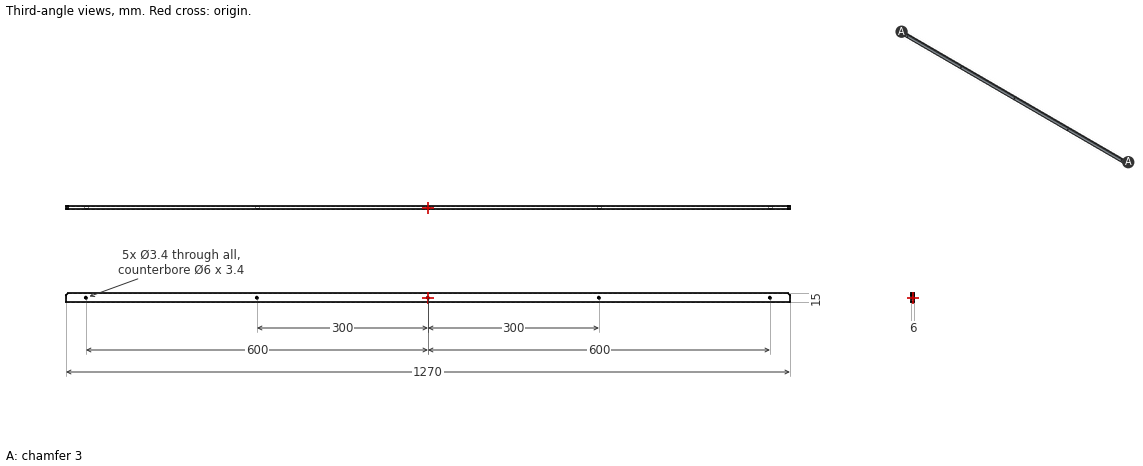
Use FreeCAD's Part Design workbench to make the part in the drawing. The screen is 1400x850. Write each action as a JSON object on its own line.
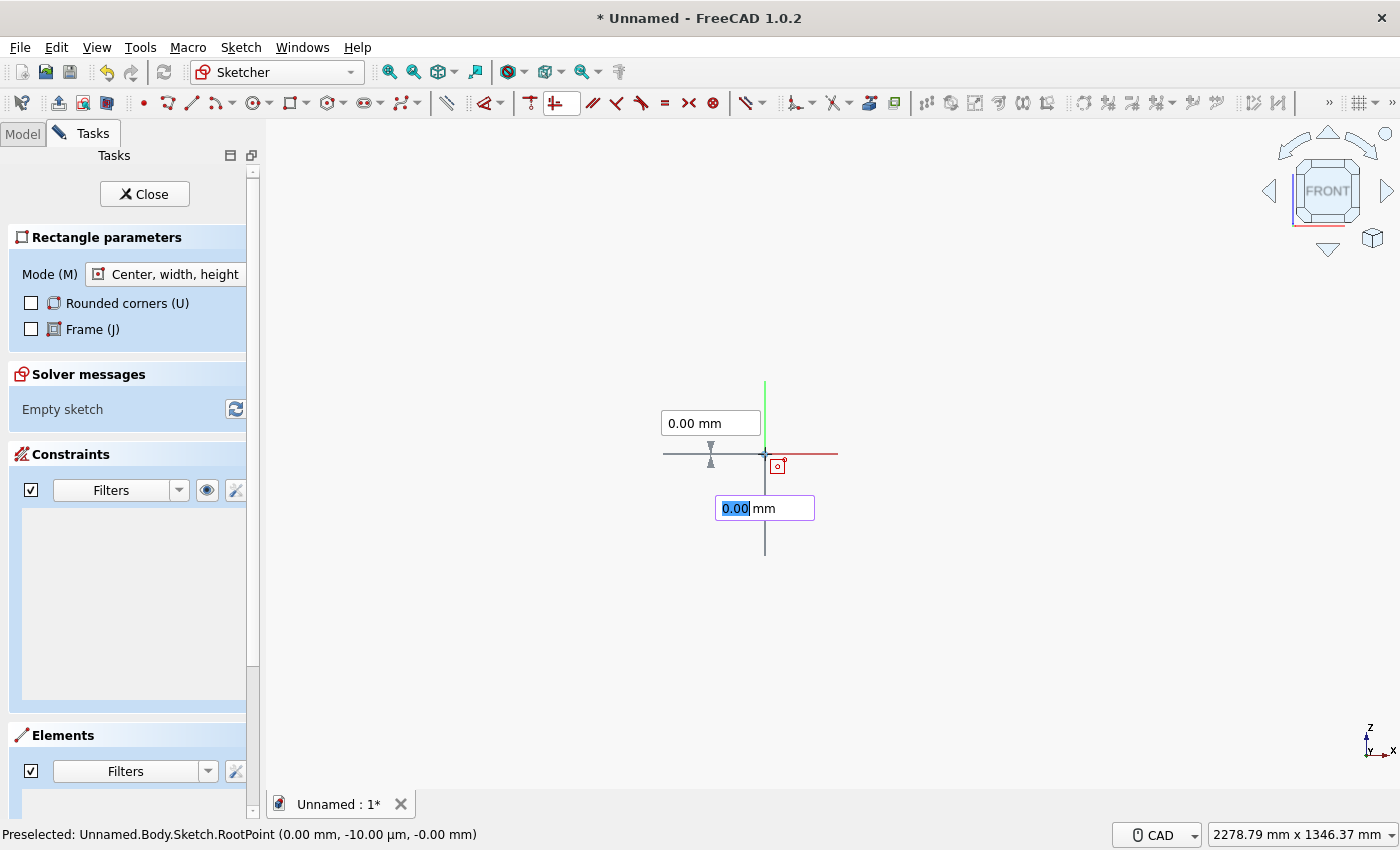
{"action": "scroll", "coordinate": [1081, 451], "scroll_direction": "up", "scroll_amount": 8}
{"action": "mouse_move", "coordinate": [1078, 448]}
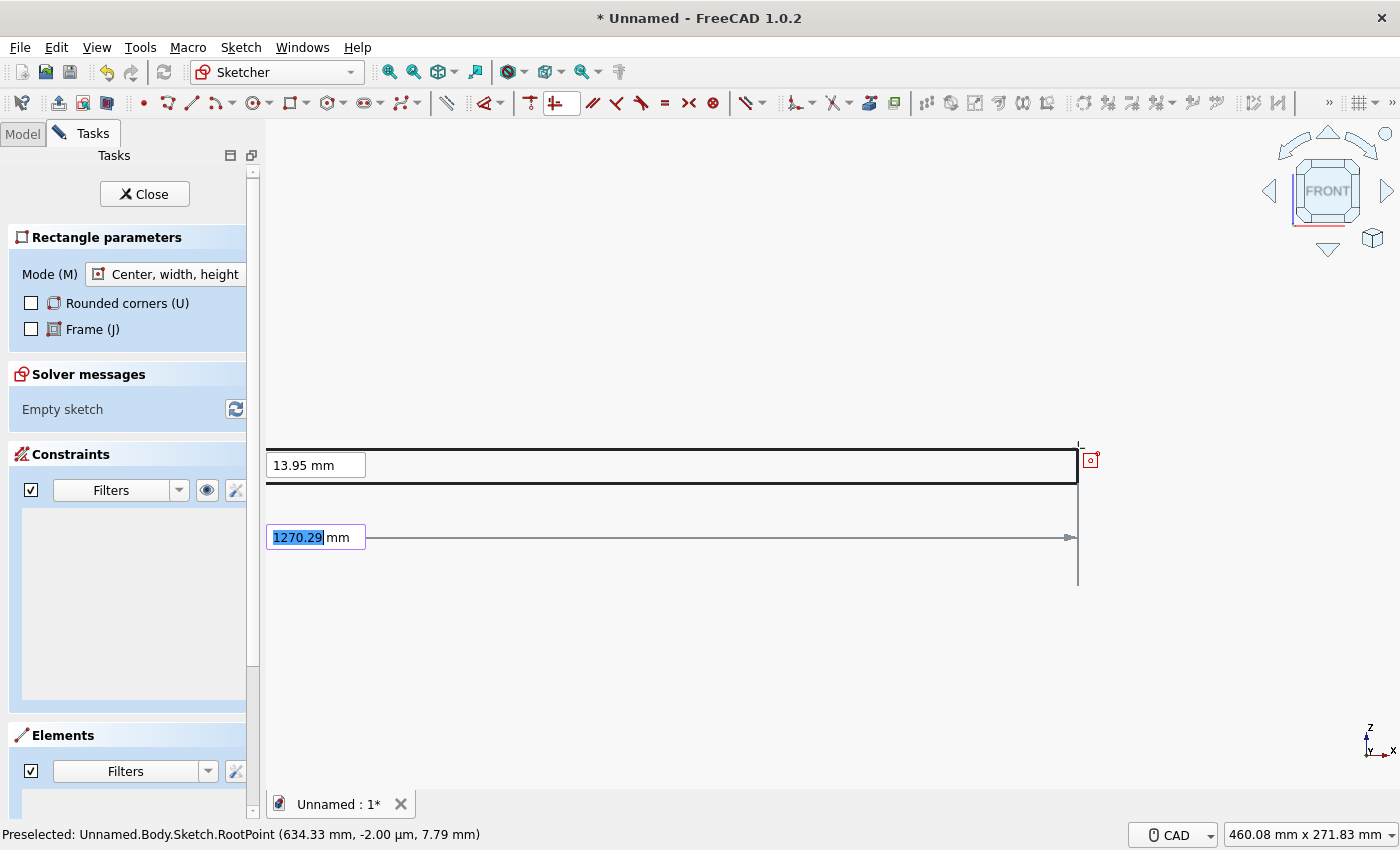
{"action": "type", "text": "1270"}
{"action": "key", "text": "Tab"}
{"action": "type", "text": "15"}
{"action": "key", "text": "Return"}
{"action": "key", "text": "Escape"}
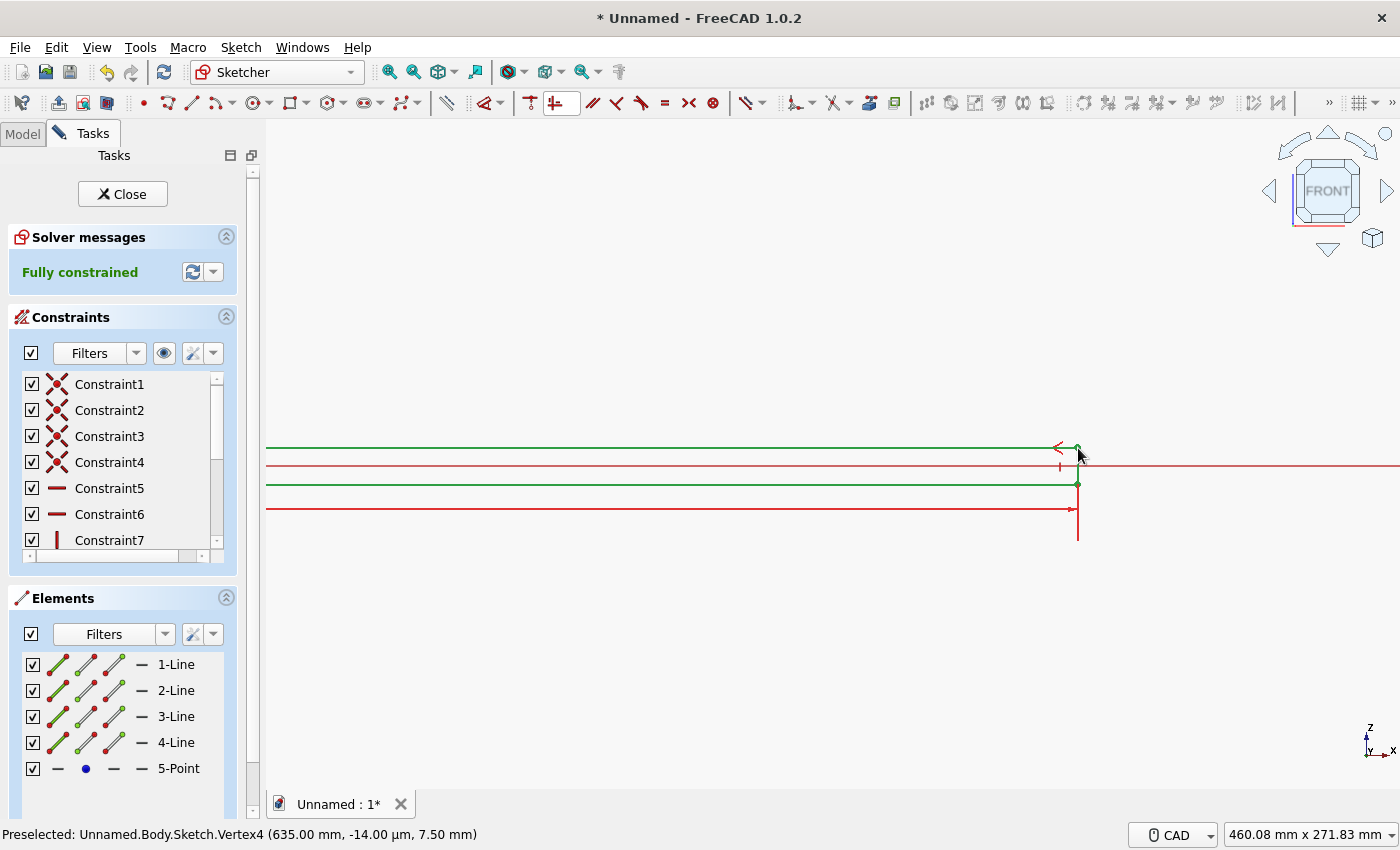
{"action": "left_click", "coordinate": [123, 194]}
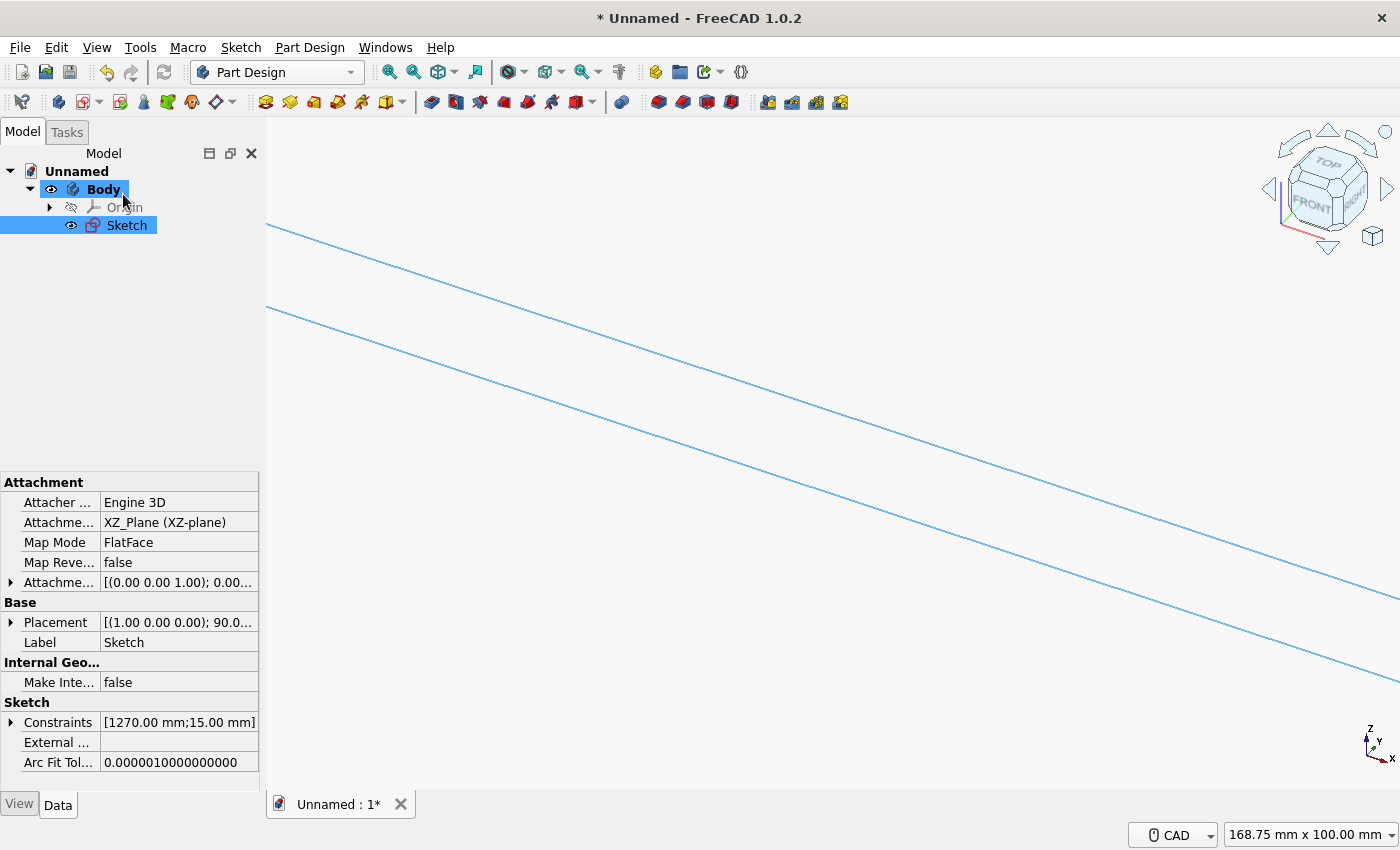
{"action": "left_click", "coordinate": [266, 102]}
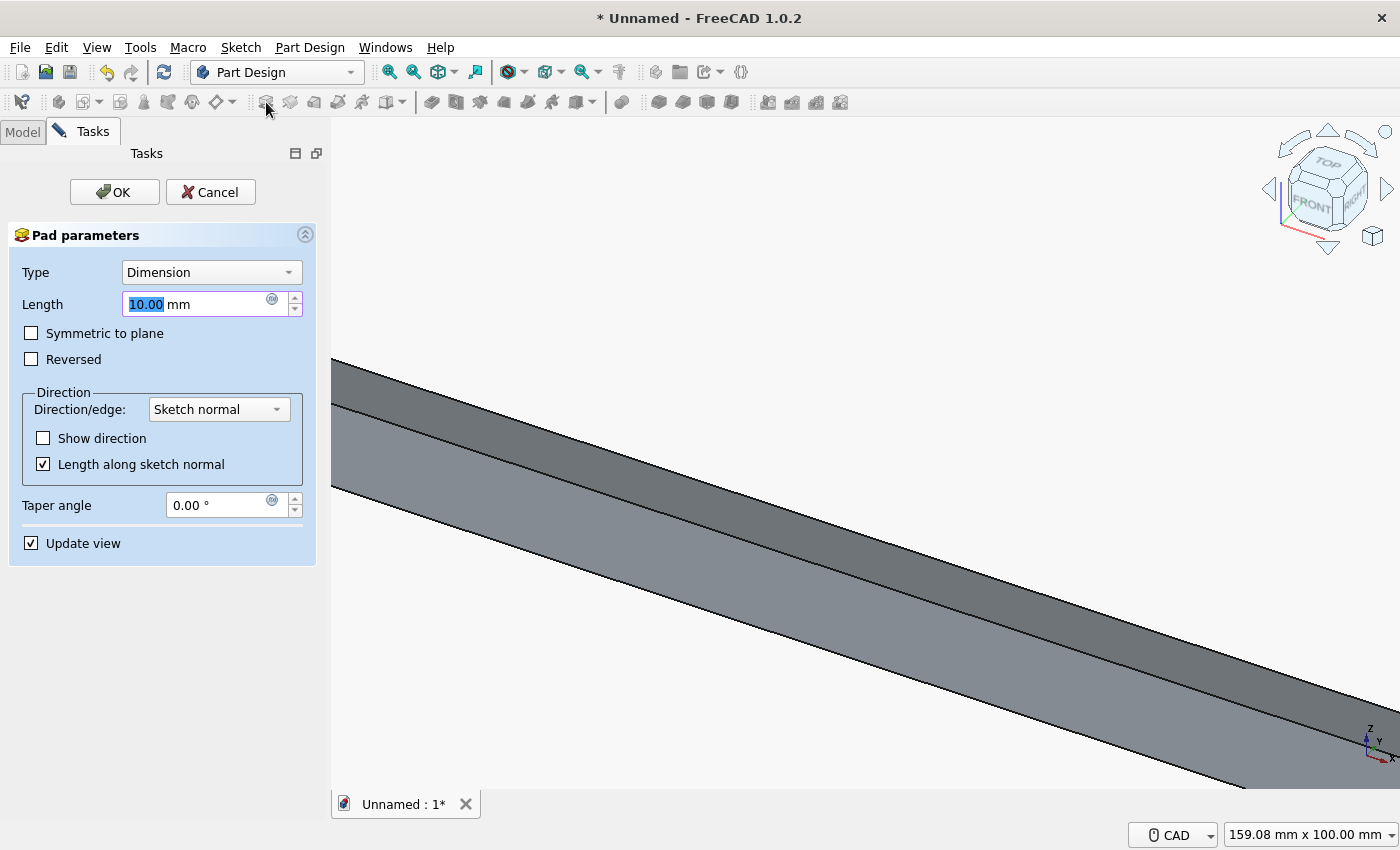
{"action": "type", "text": "6"}
{"action": "key", "text": "Tab"}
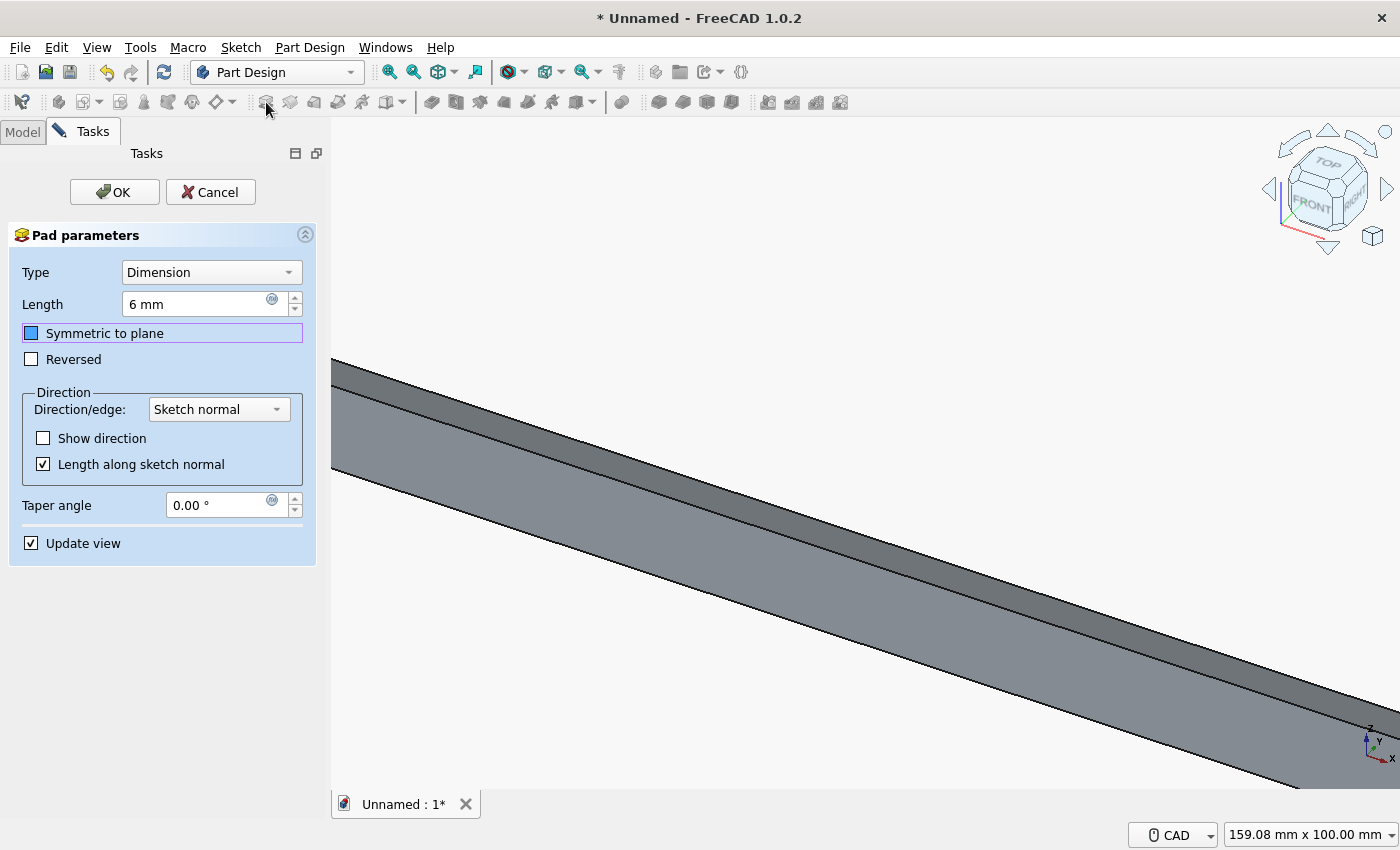
{"action": "left_click", "coordinate": [30, 333]}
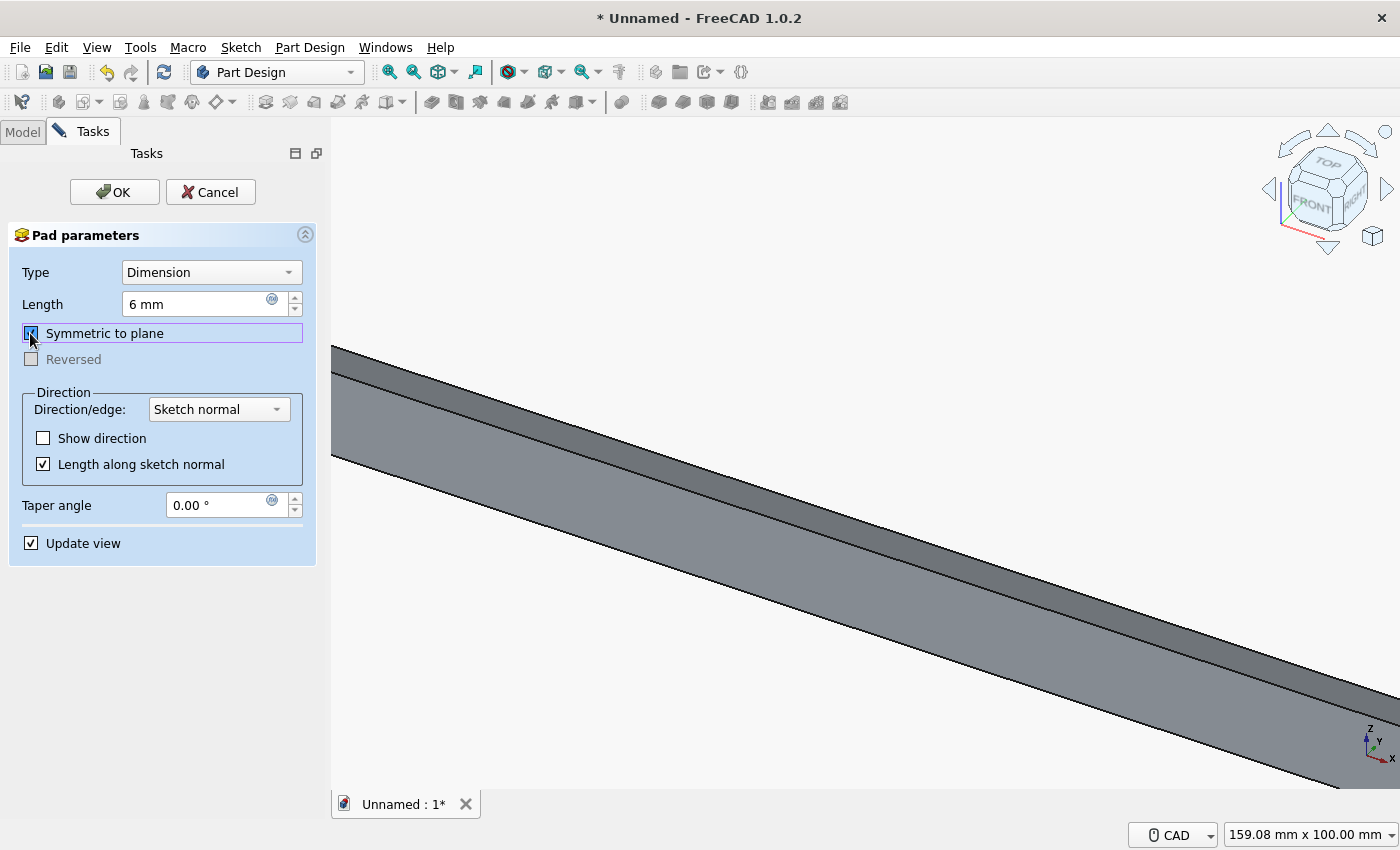
{"action": "left_click", "coordinate": [115, 192]}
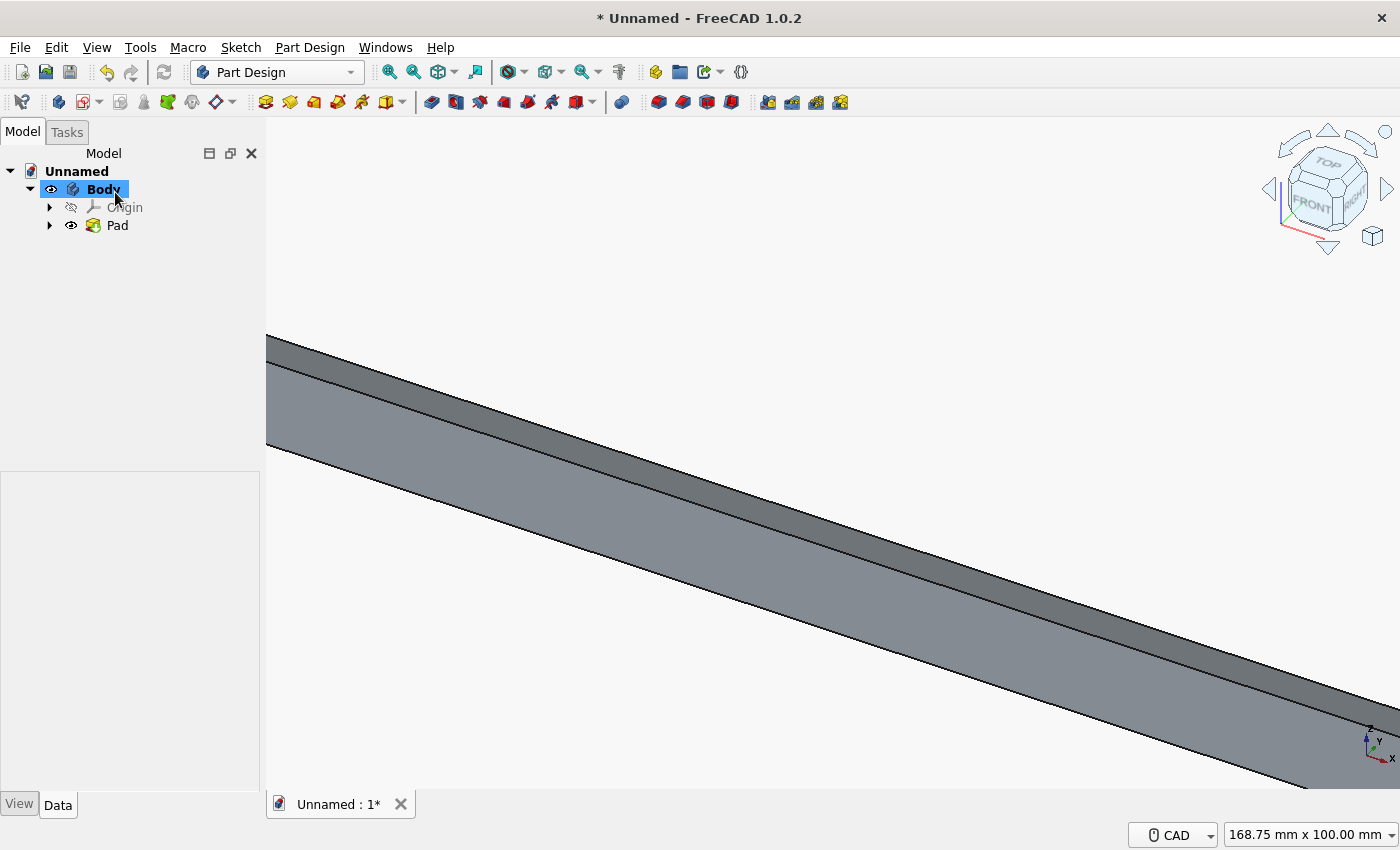
{"action": "key", "text": "v f"}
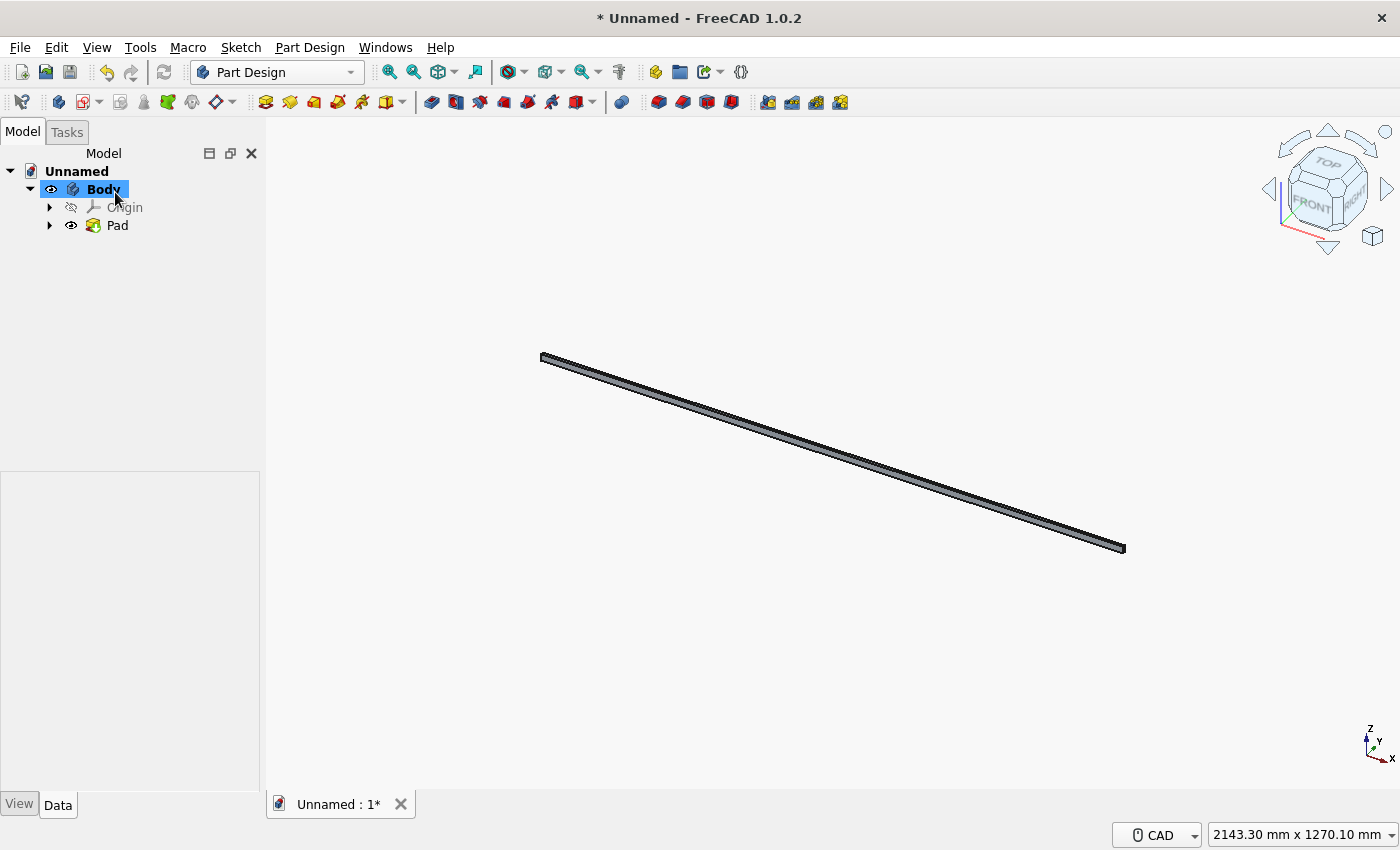
{"action": "scroll", "coordinate": [1124, 545], "scroll_direction": "up", "scroll_amount": 13}